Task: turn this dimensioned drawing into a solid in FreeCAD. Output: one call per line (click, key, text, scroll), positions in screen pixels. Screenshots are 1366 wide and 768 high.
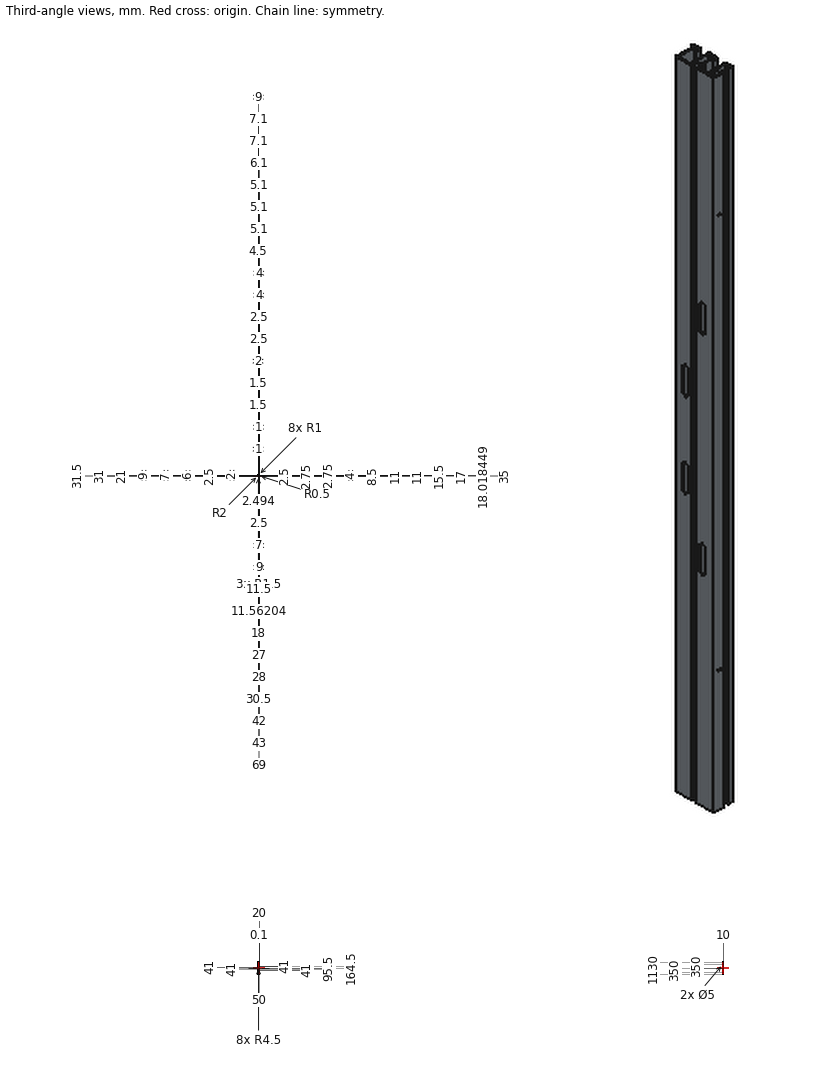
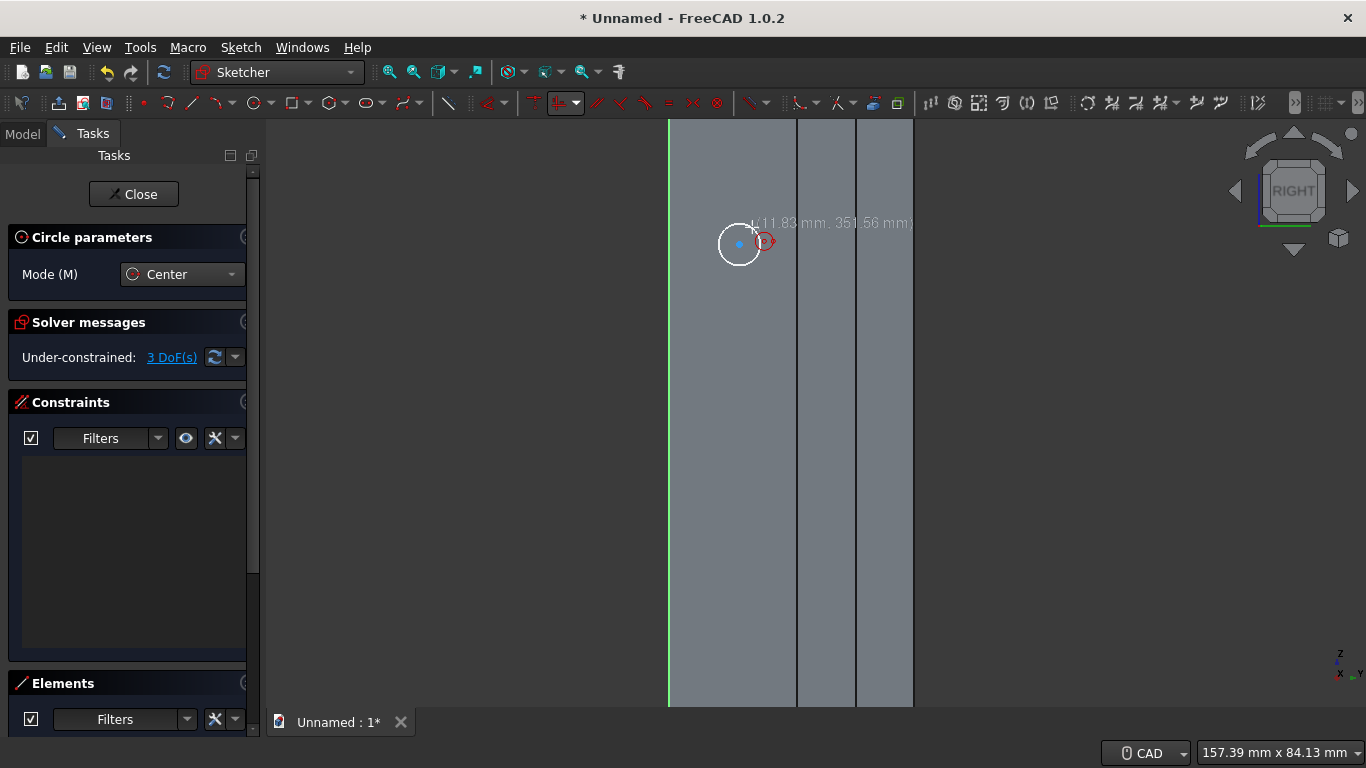
scroll(750, 231, down, 13)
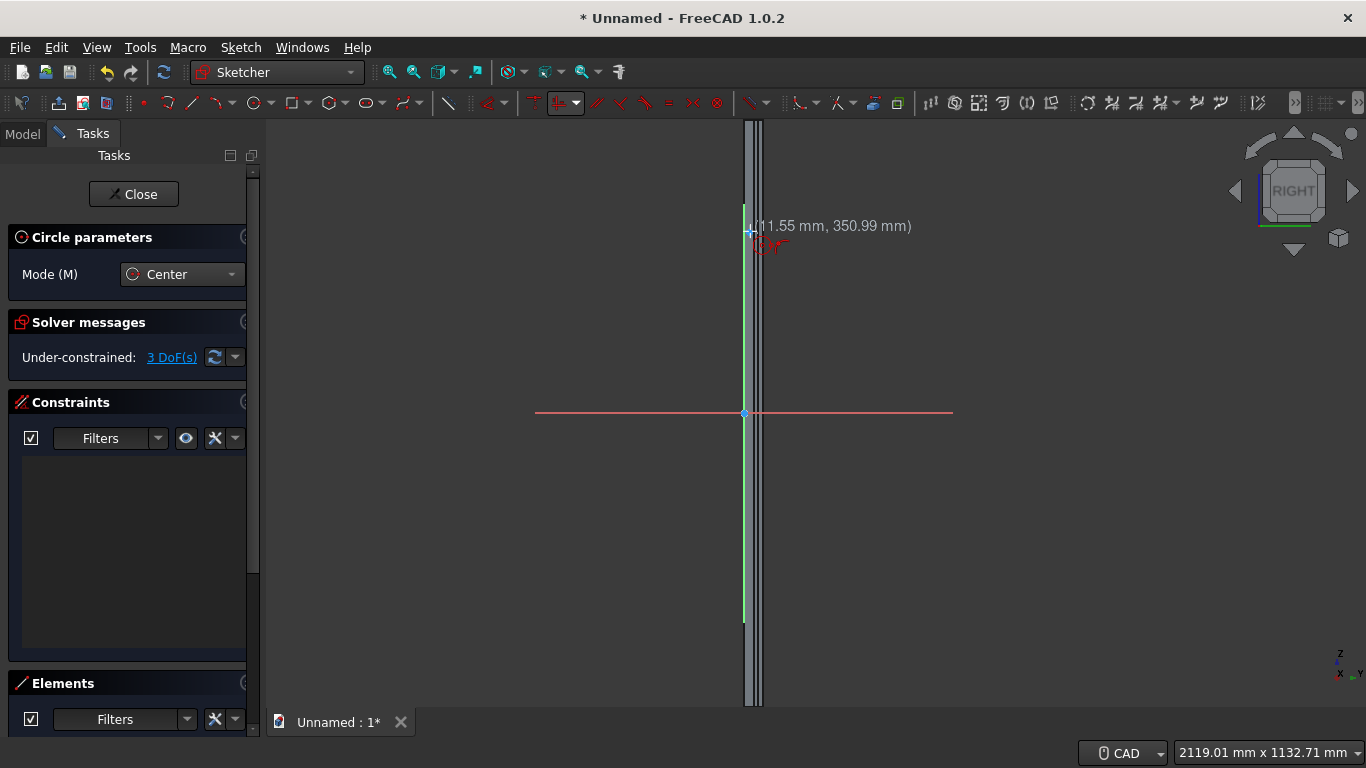
scroll(750, 595, up, 15)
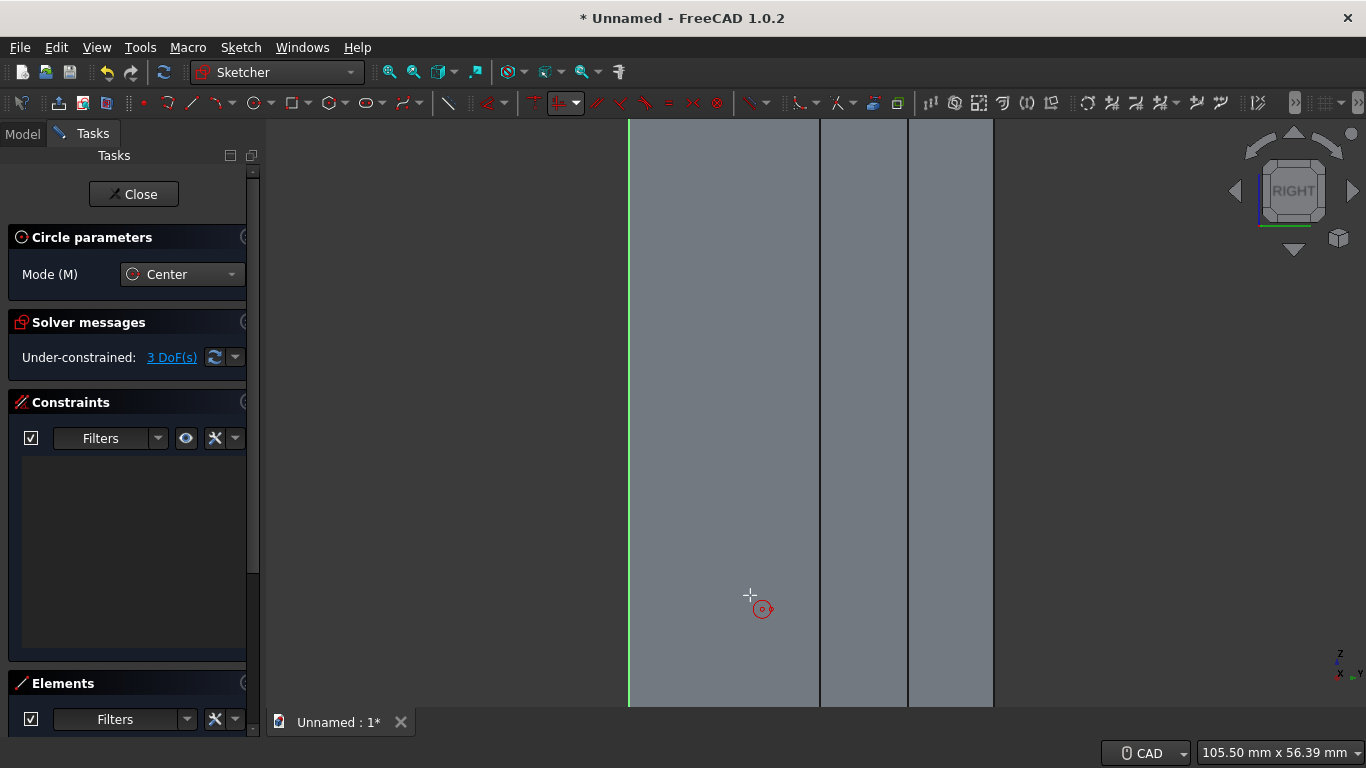
scroll(750, 595, down, 15)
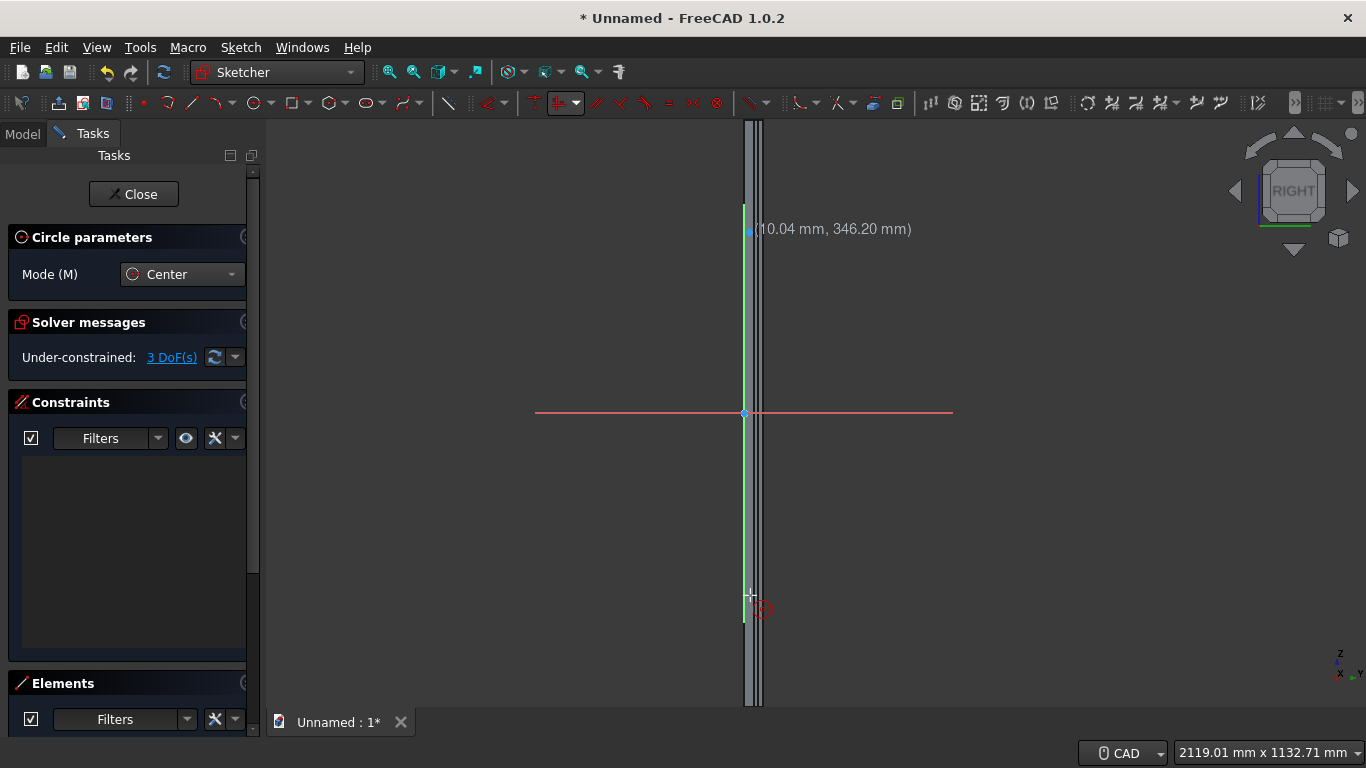
scroll(750, 595, up, 6)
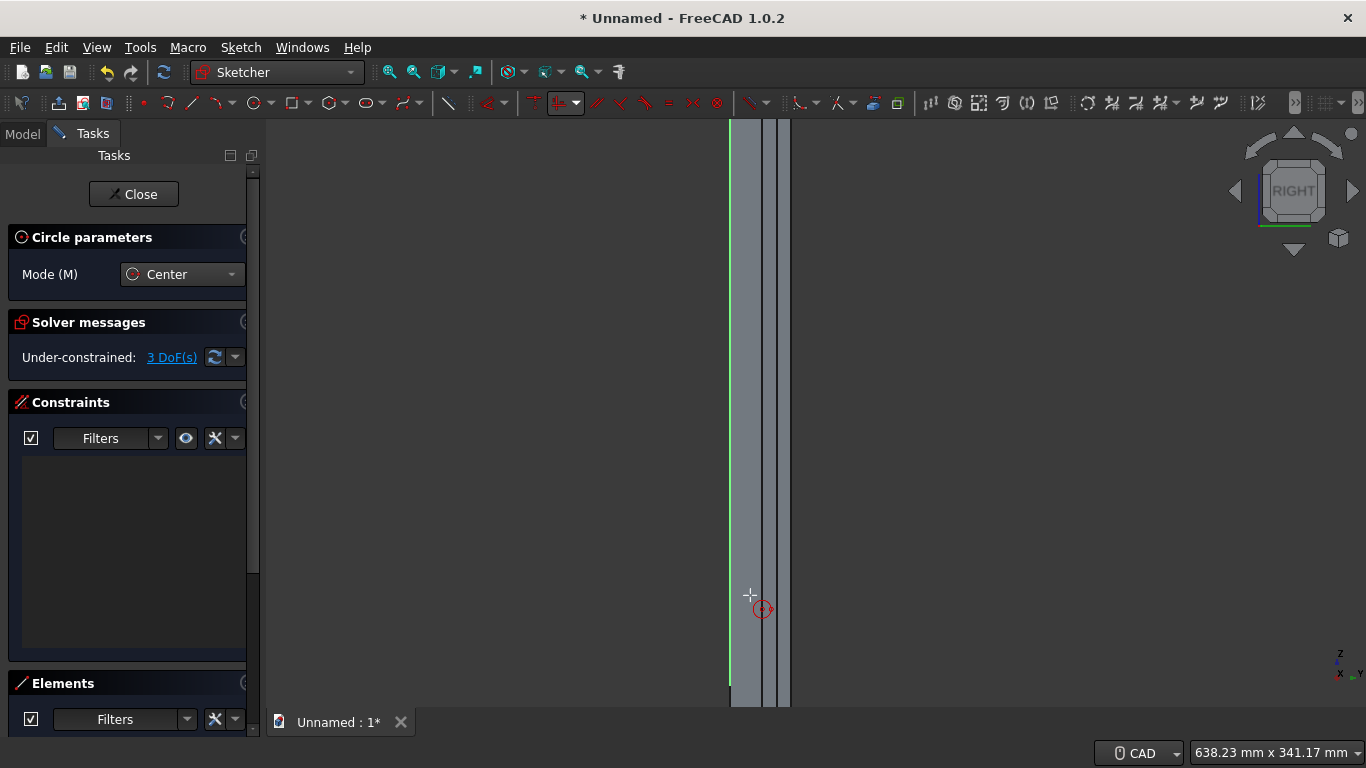
click(748, 594)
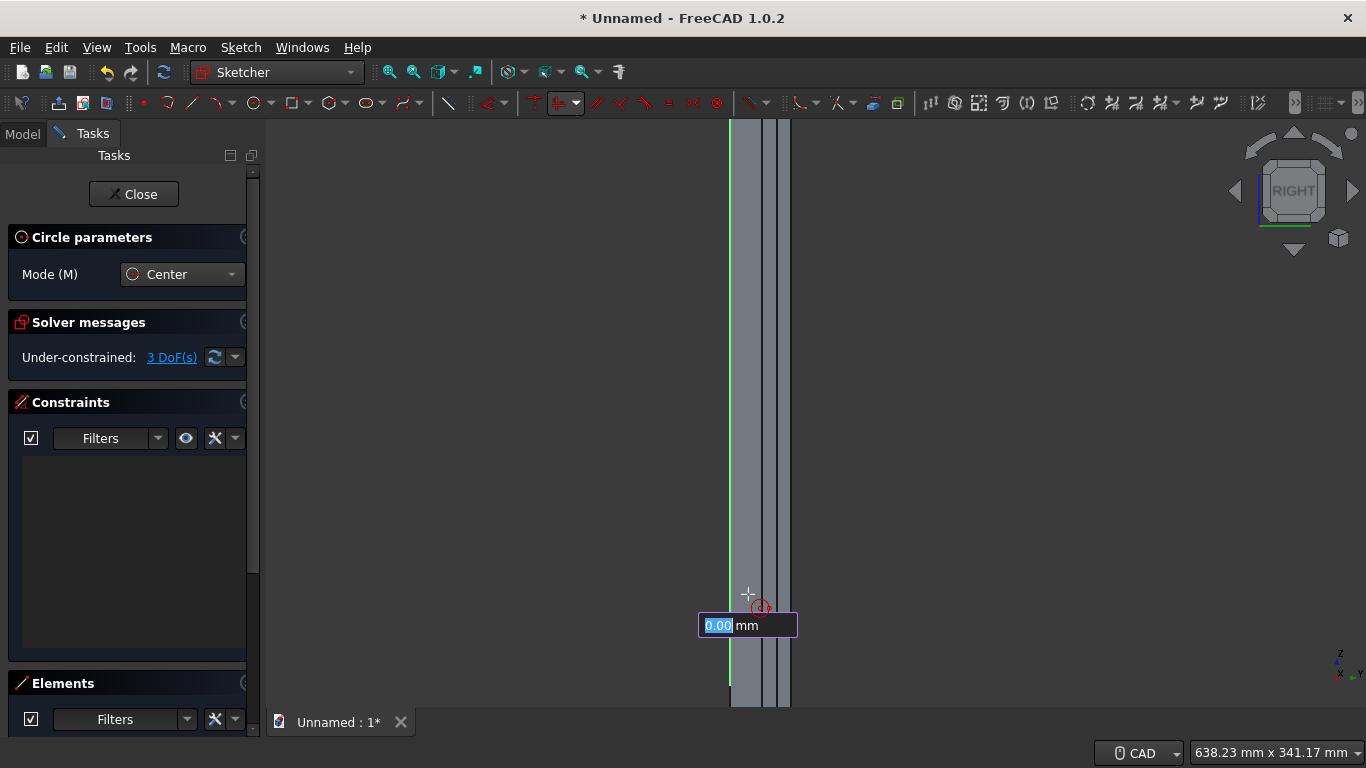
scroll(751, 591, up, 7)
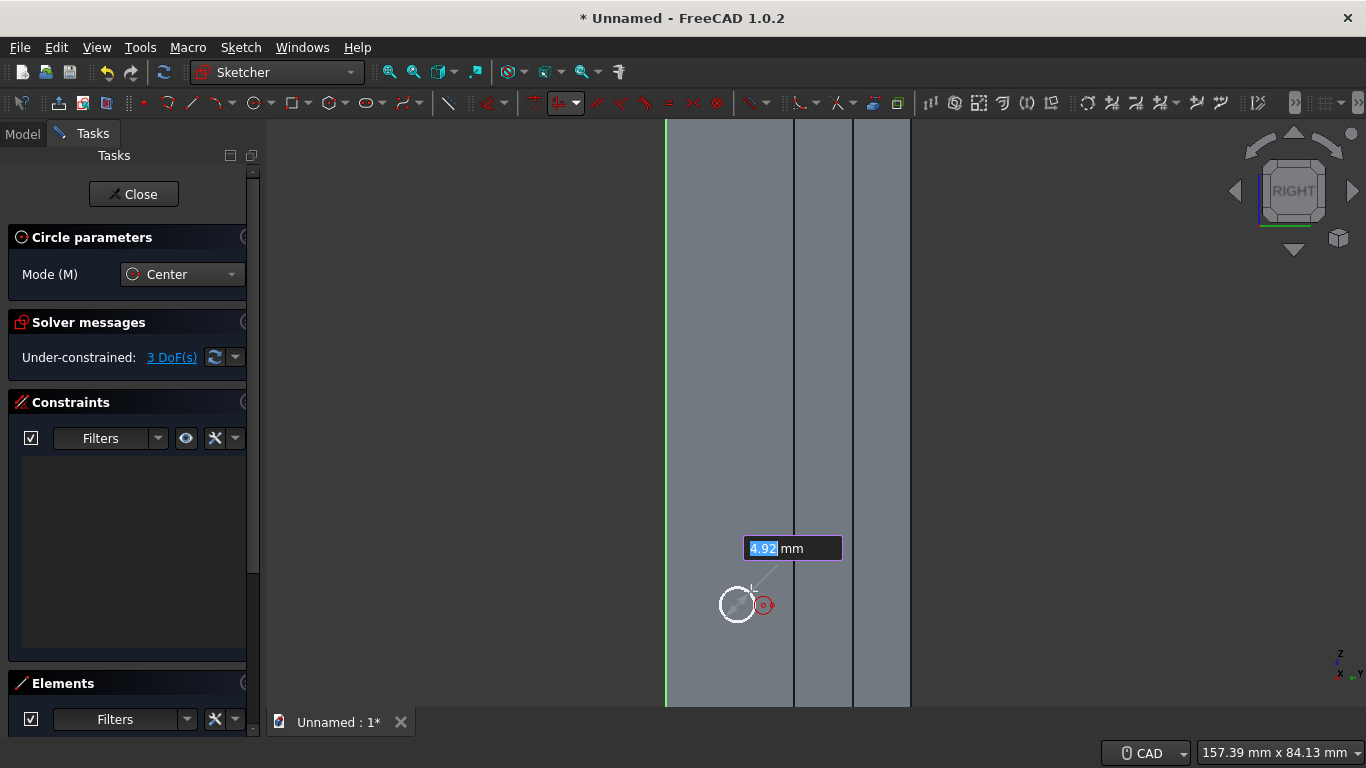
click(748, 587)
key(Escape)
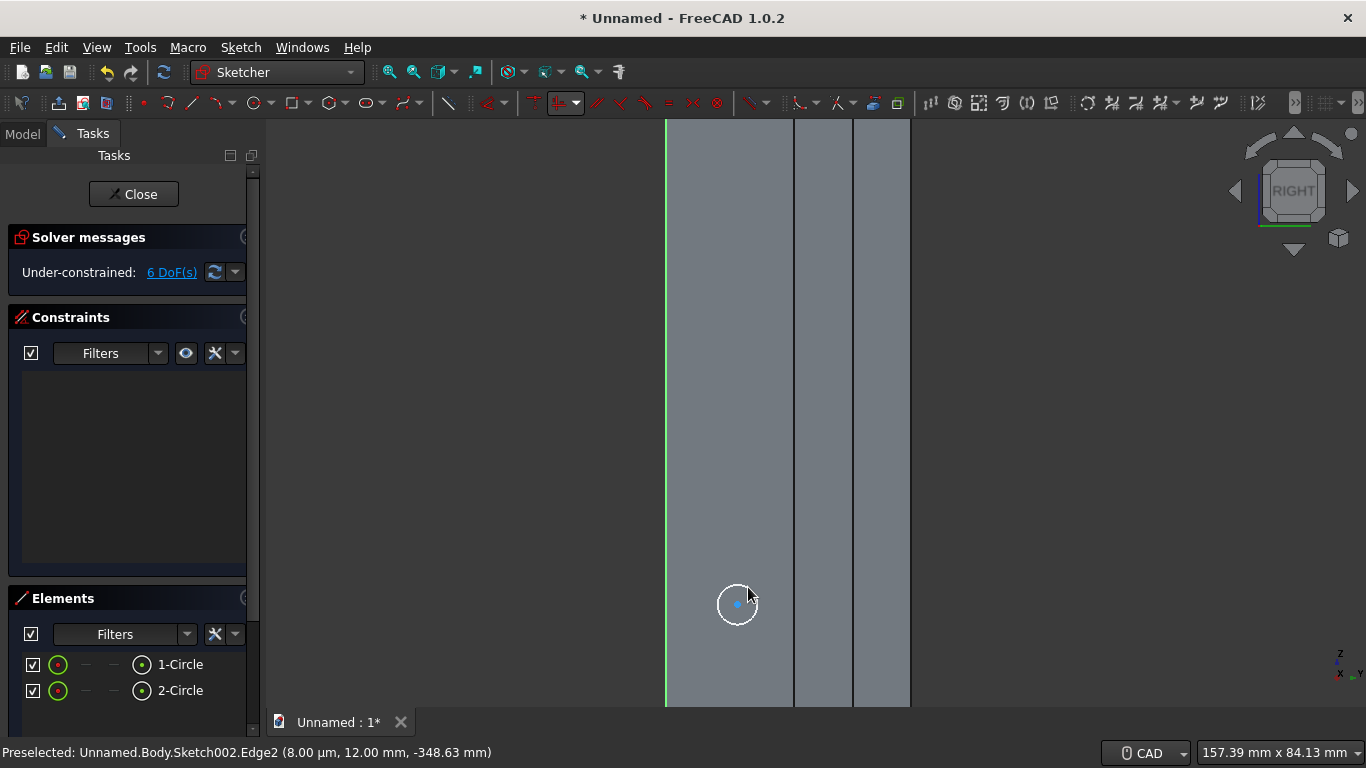
scroll(751, 594, down, 13)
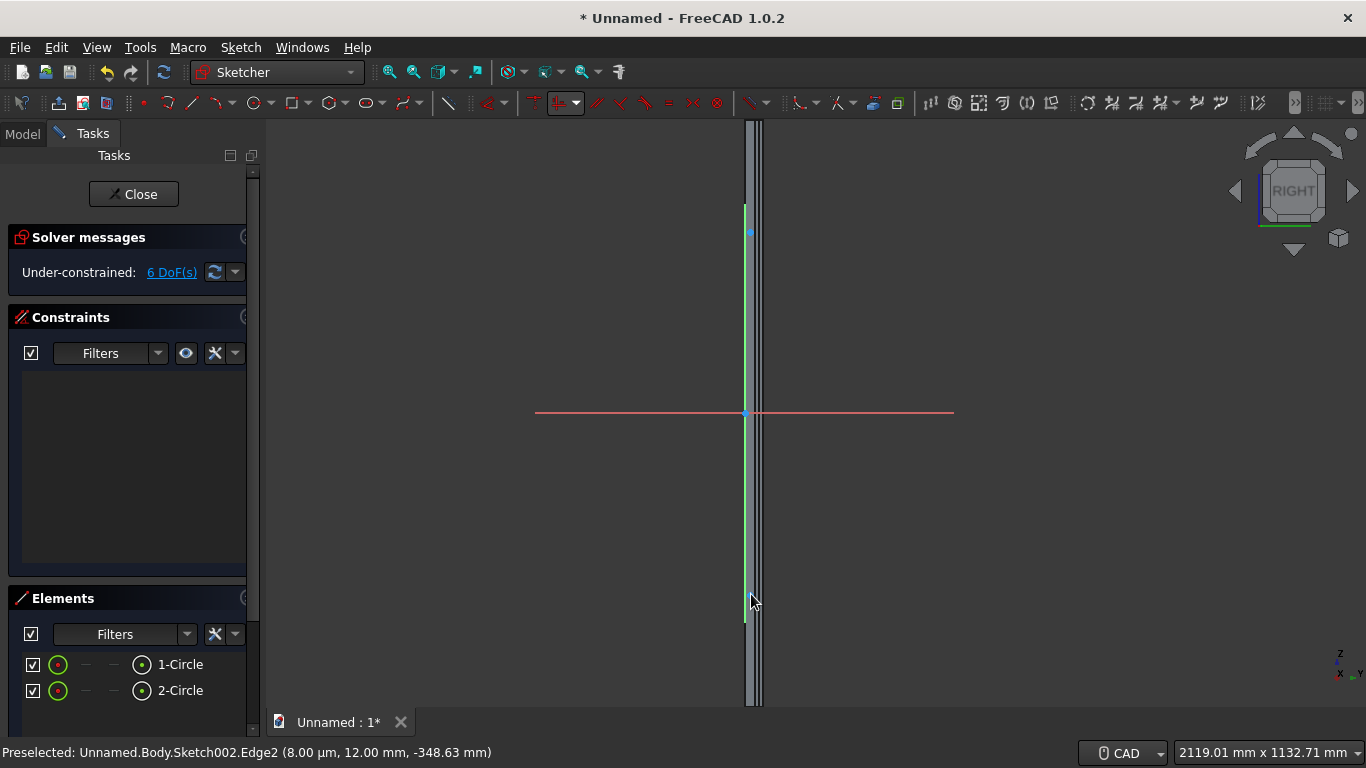
scroll(751, 231, up, 11)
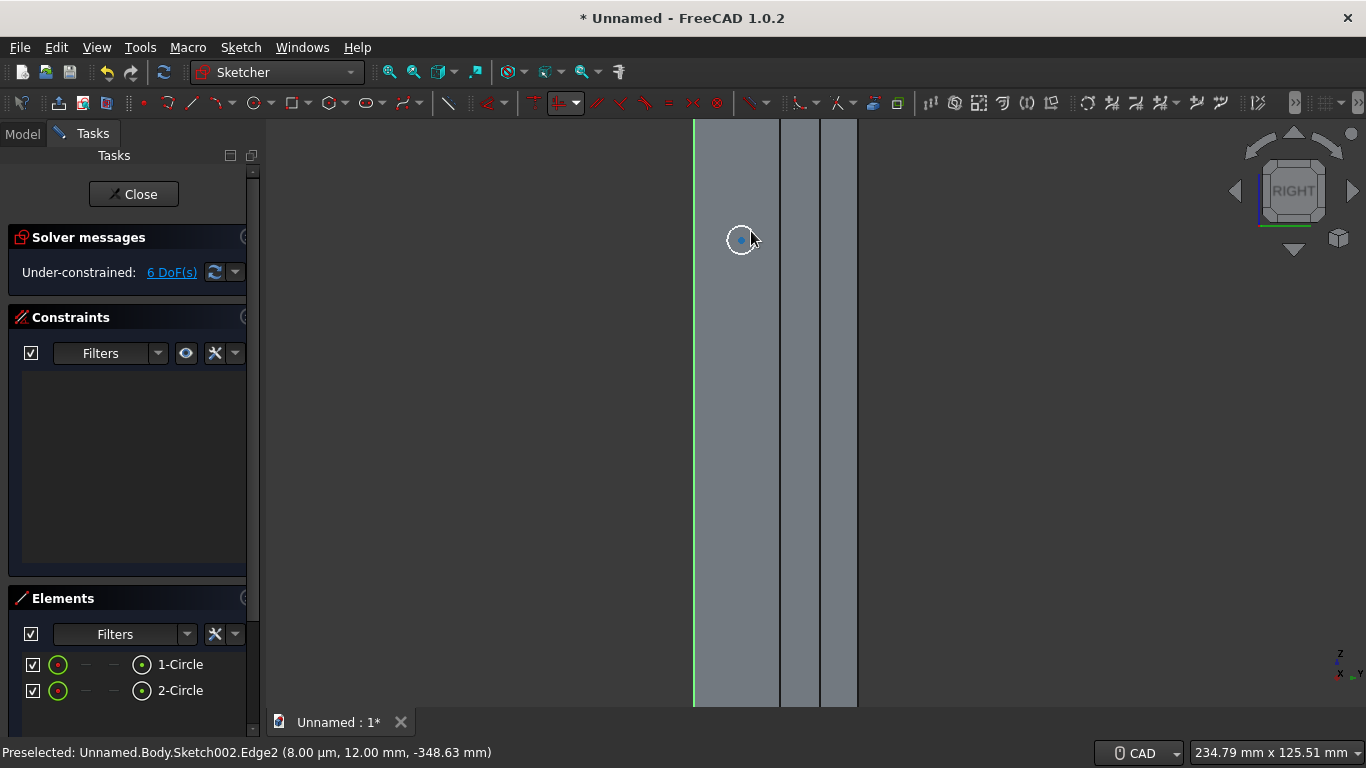
click(751, 230)